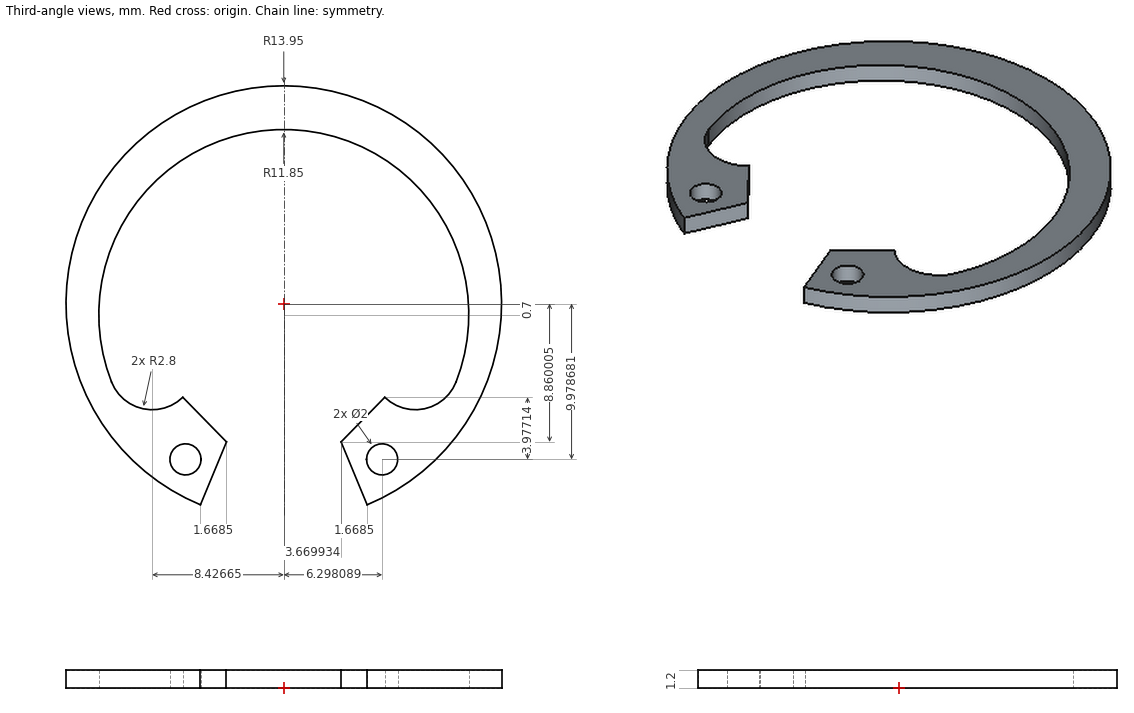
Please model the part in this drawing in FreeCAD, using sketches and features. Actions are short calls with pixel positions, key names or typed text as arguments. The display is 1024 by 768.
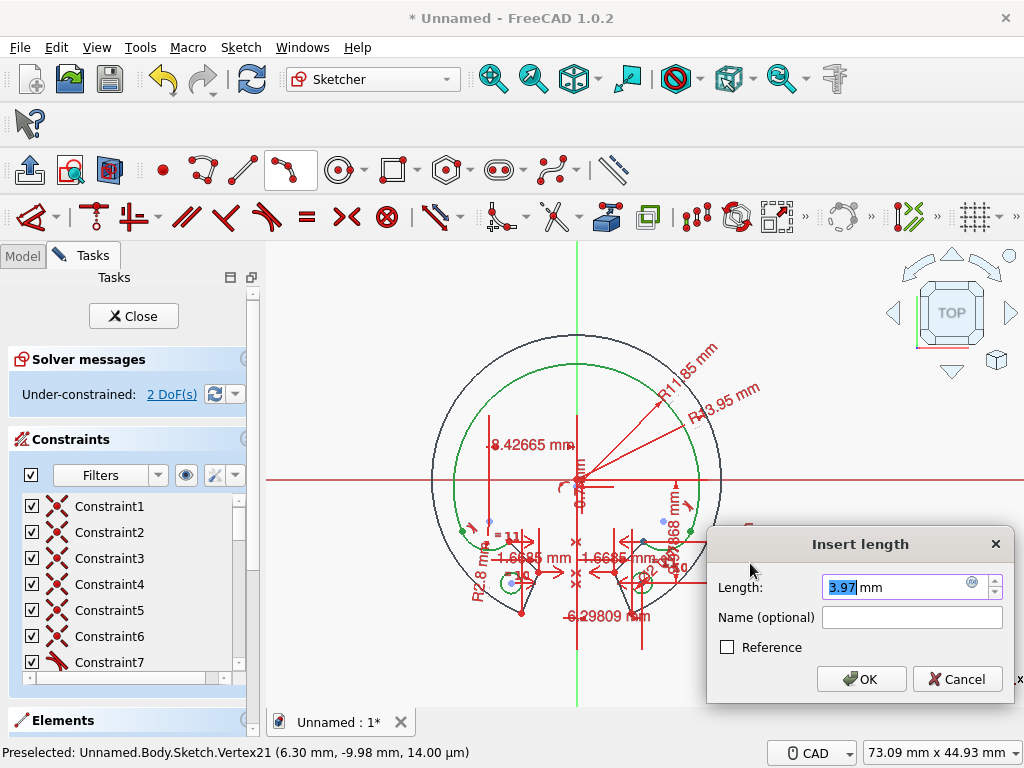
text(3.97714)
key(Return)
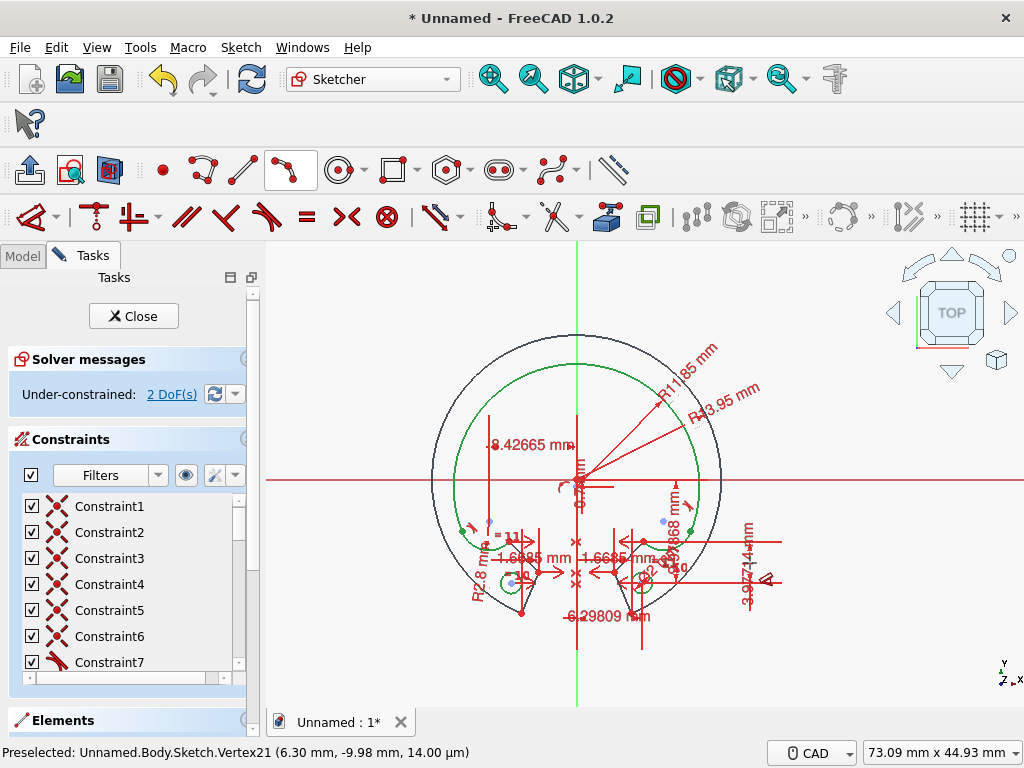
click(614, 572)
click(604, 446)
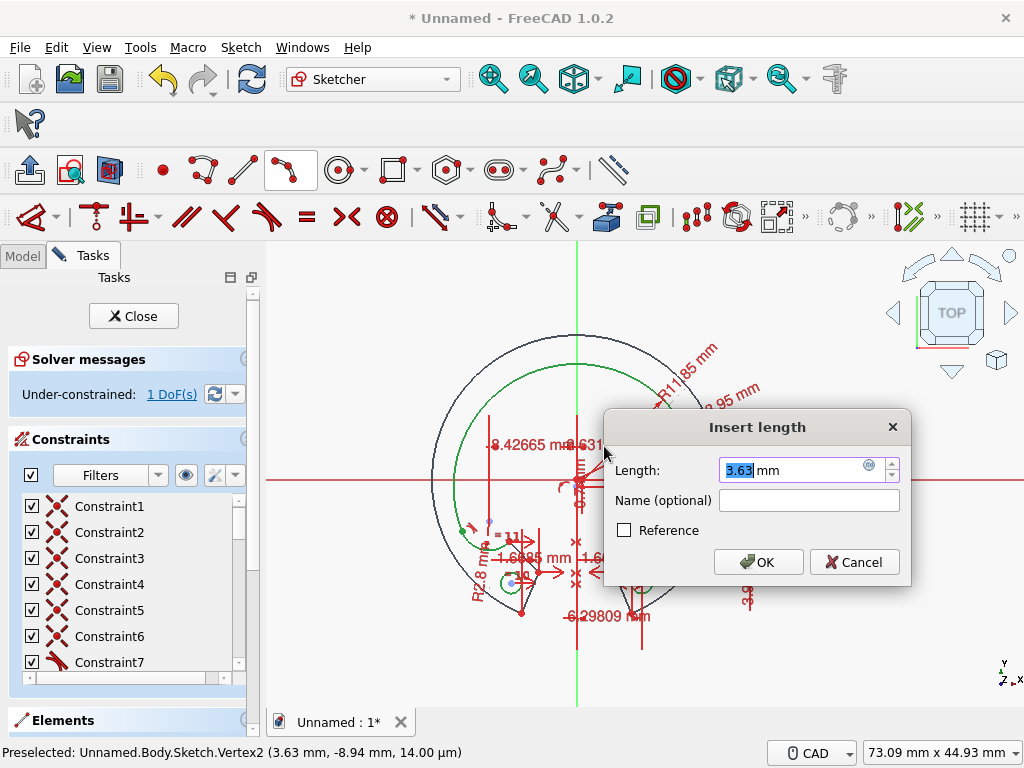
text(3.669934)
key(Return)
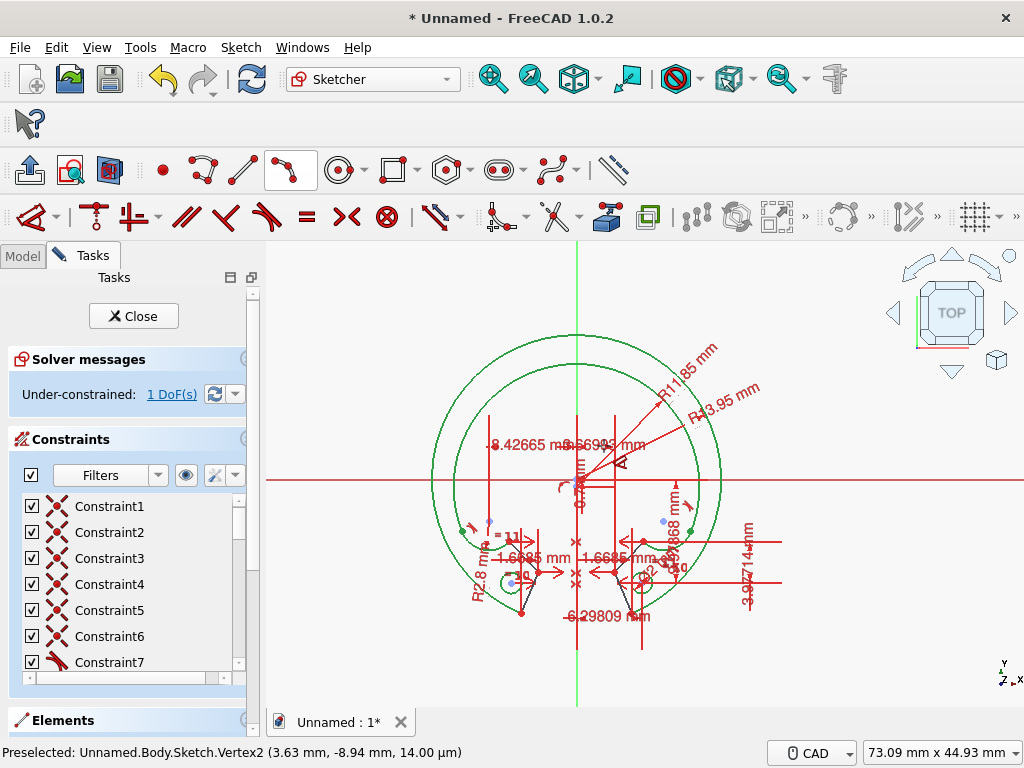
click(615, 572)
click(649, 505)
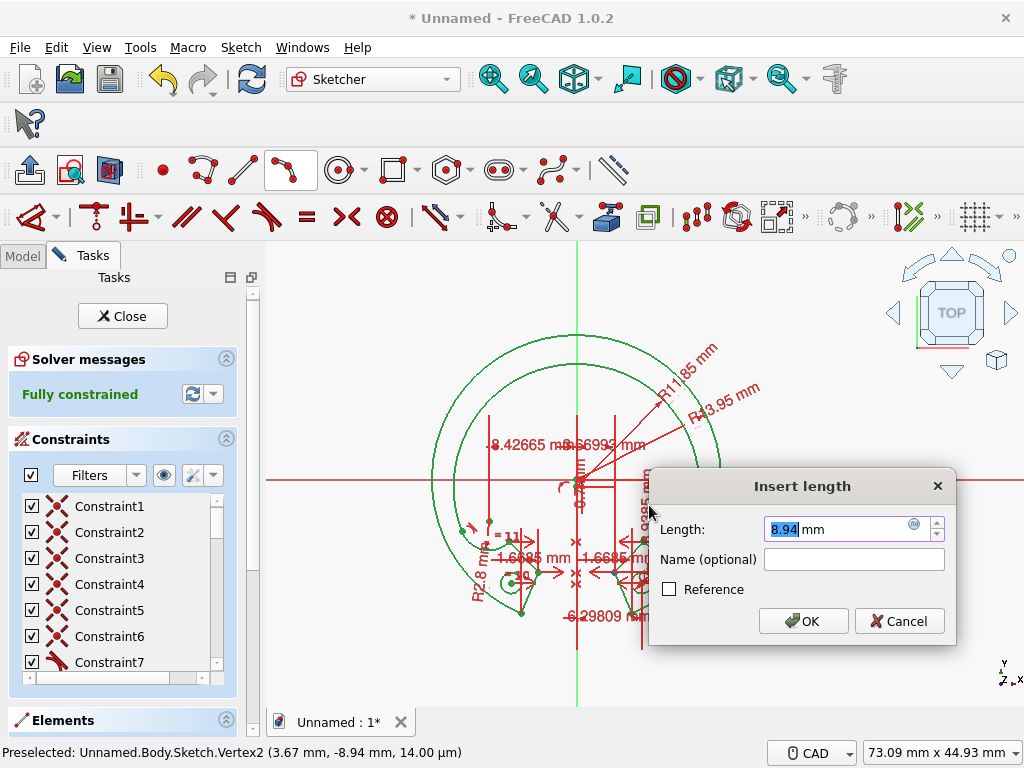
text(8.860005)
key(Return)
key(Escape)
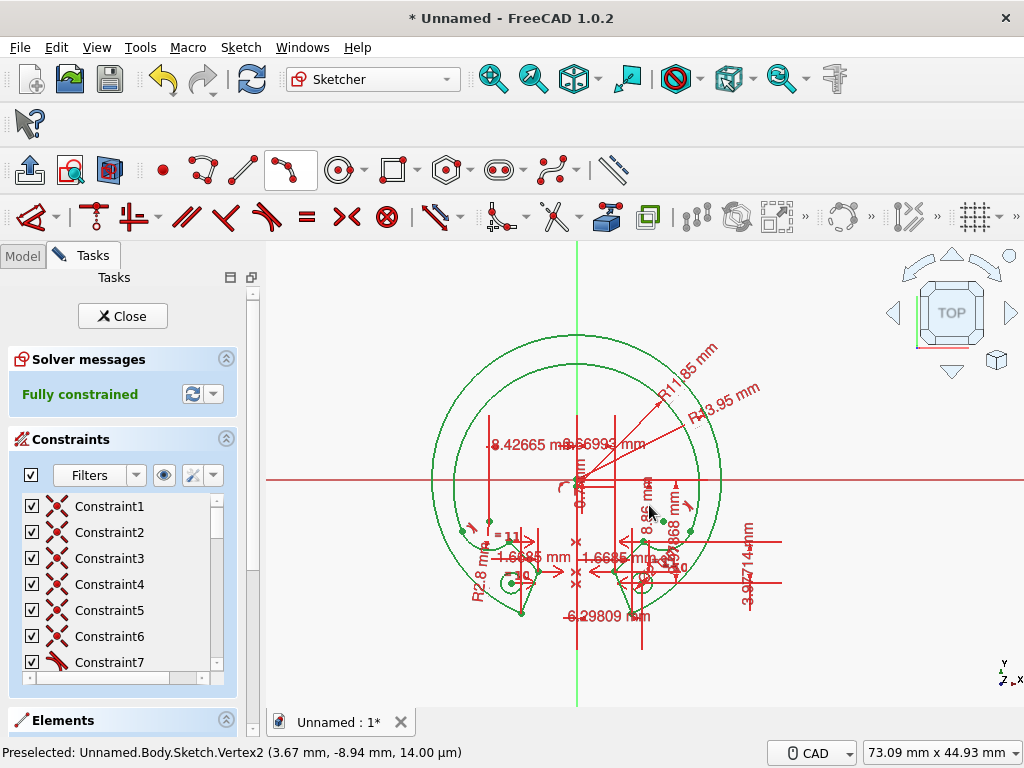
click(123, 316)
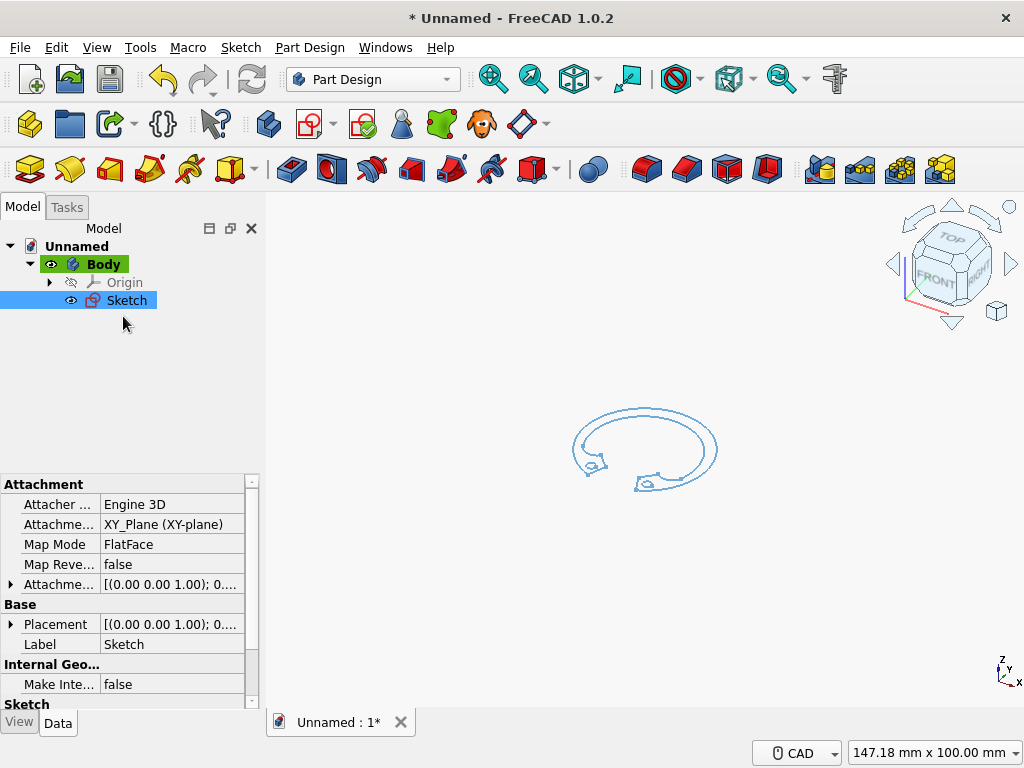
click(30, 170)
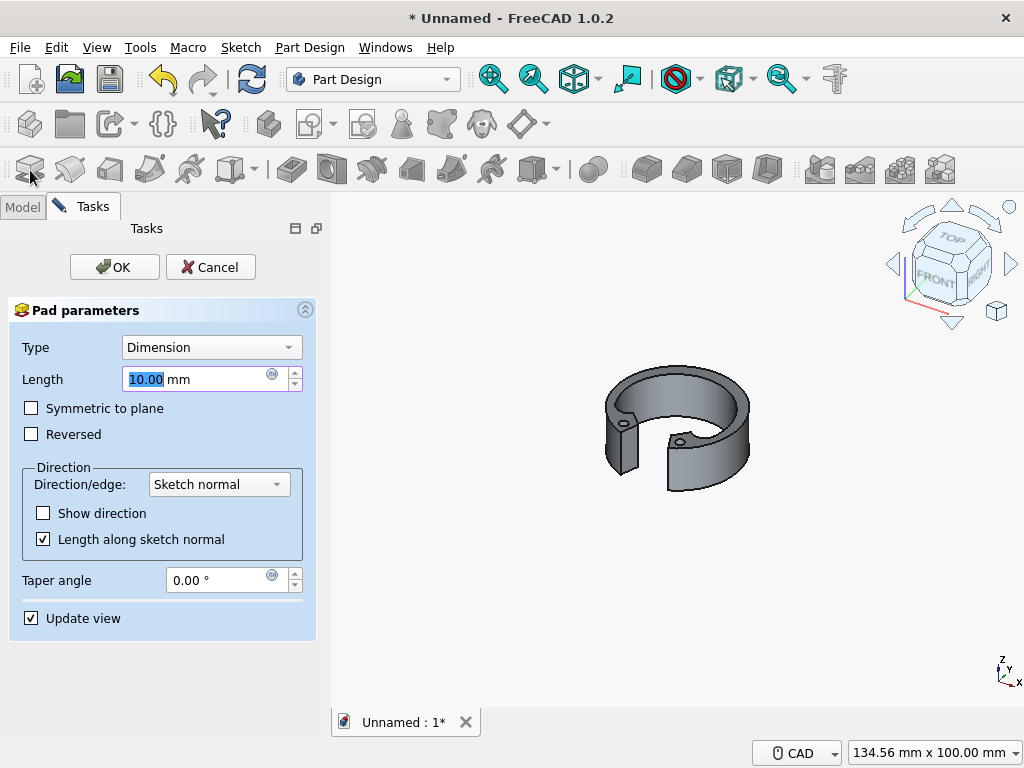
text(1.2)
key(Tab)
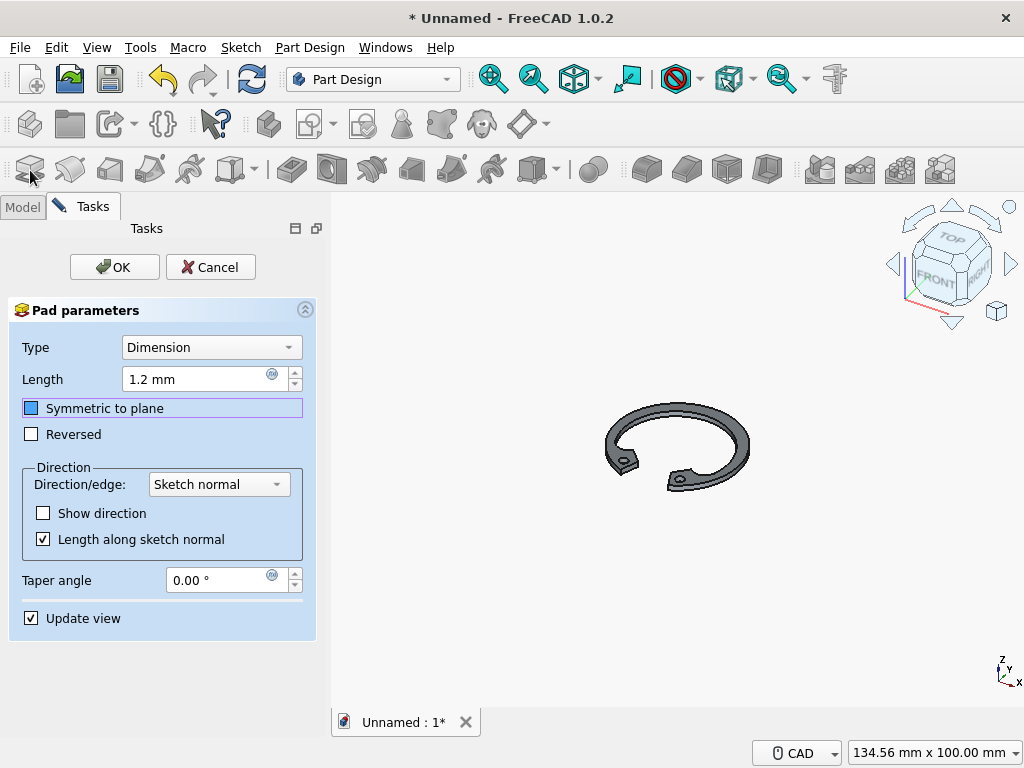
click(115, 267)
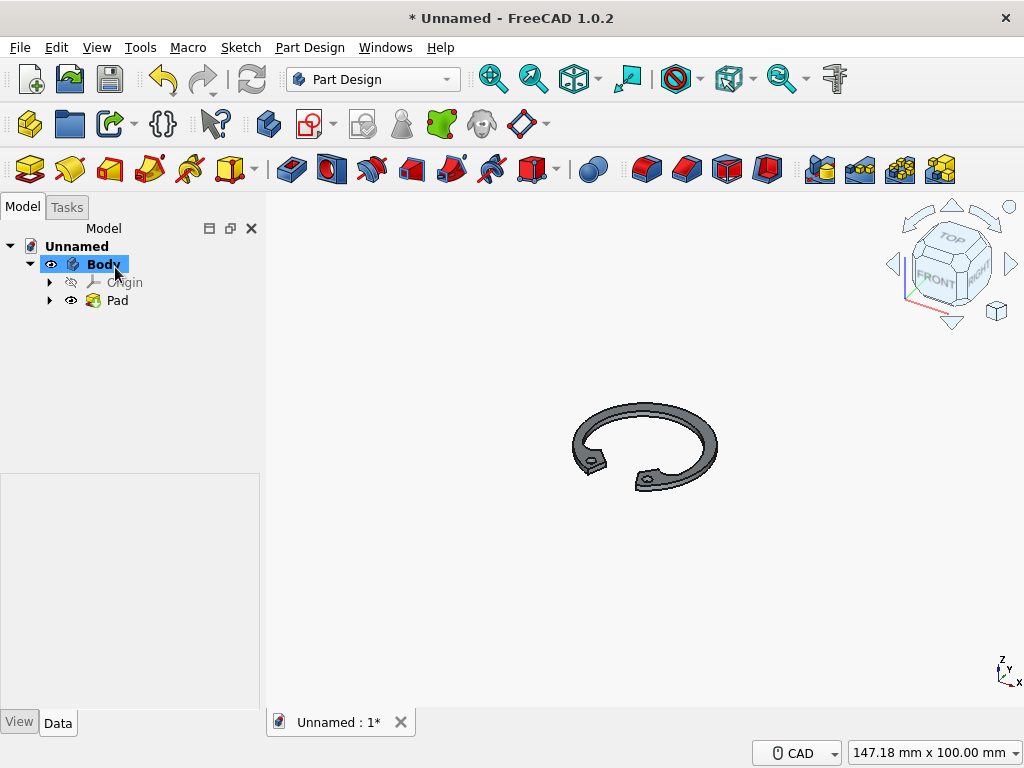
key(0)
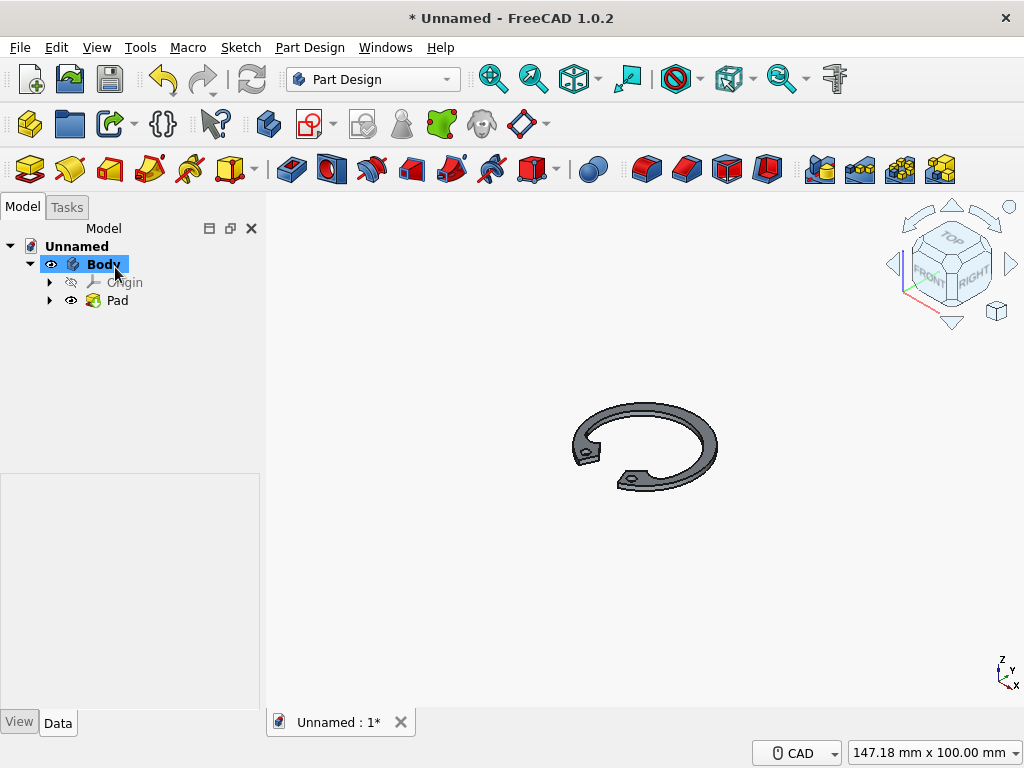
click(494, 80)